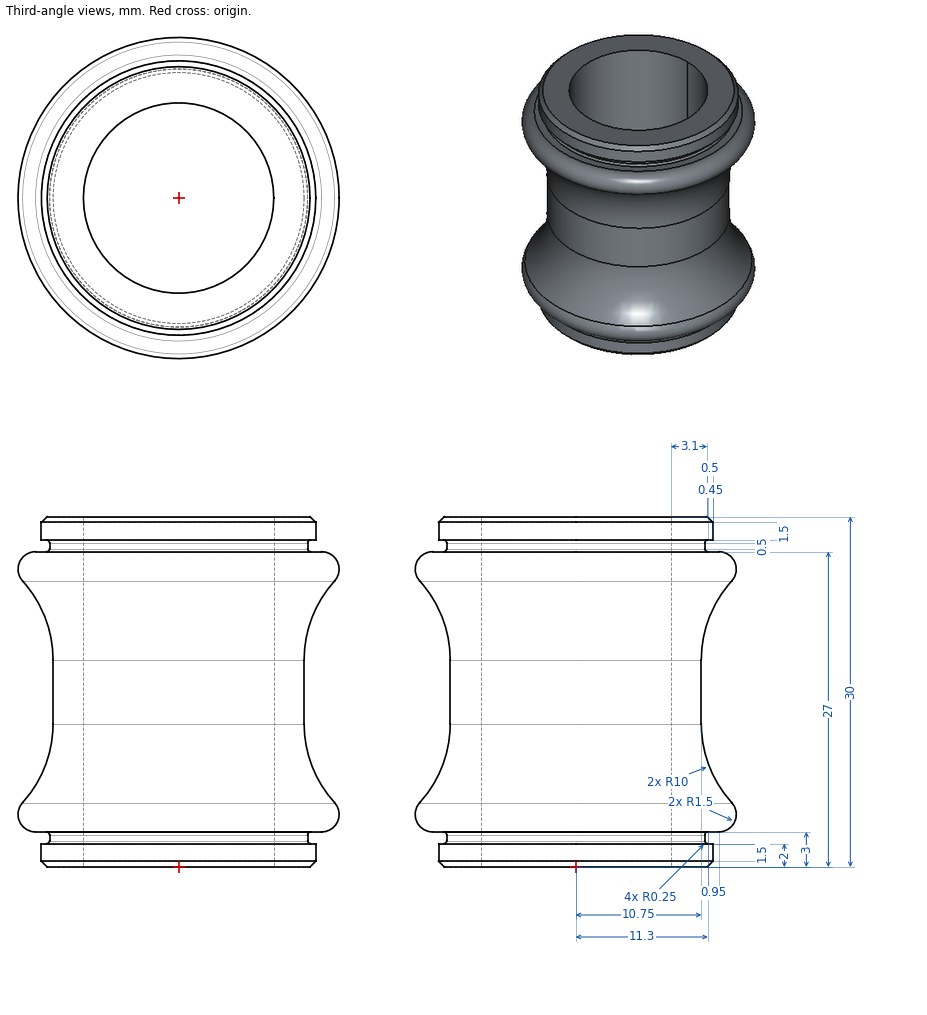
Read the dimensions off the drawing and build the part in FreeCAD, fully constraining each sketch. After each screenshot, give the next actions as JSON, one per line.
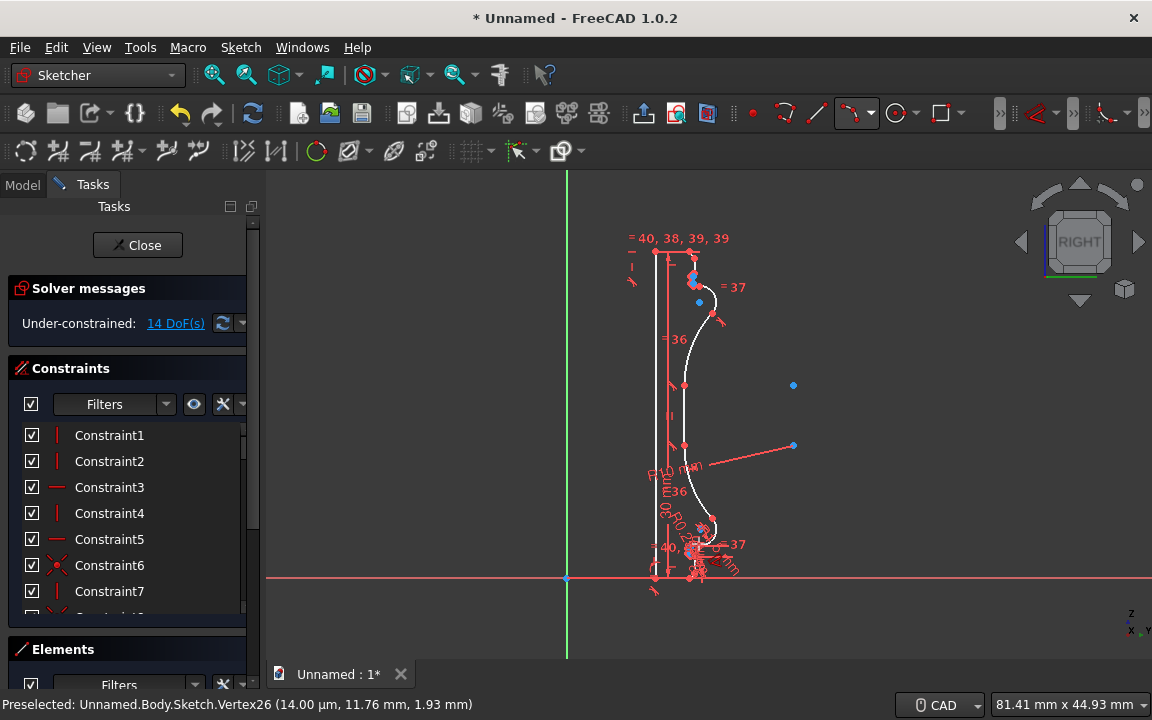
{"action": "scroll", "coordinate": [691, 281], "scroll_direction": "up", "scroll_amount": 10}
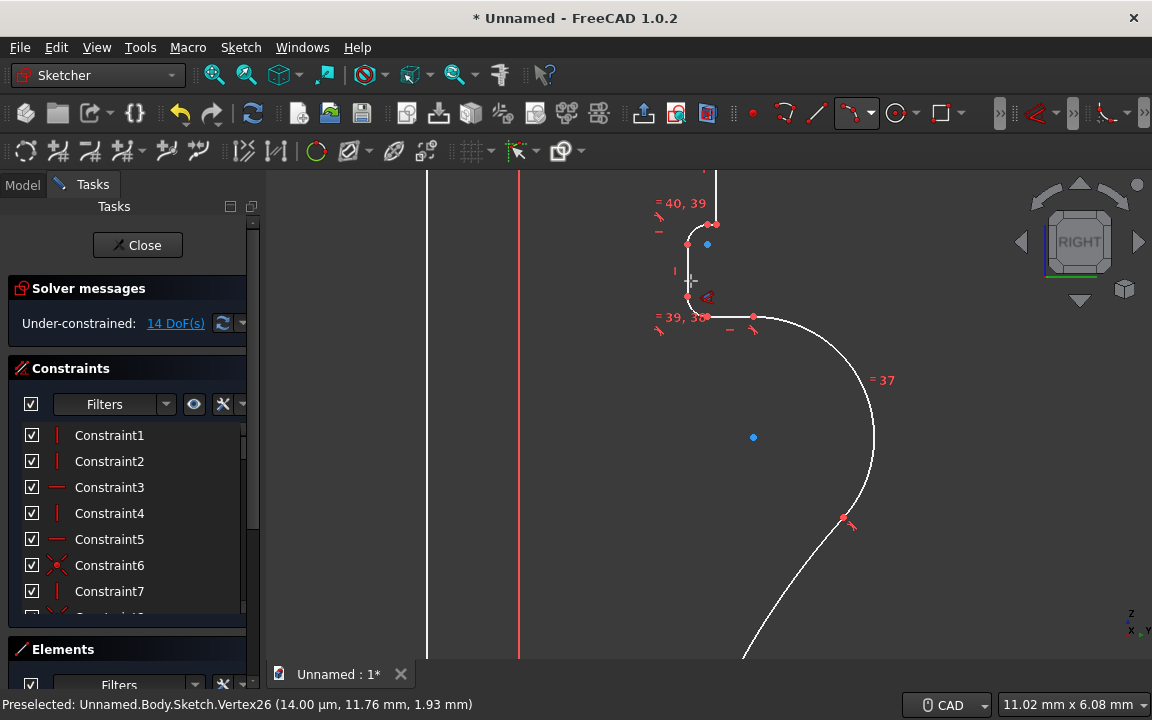
{"action": "left_click", "coordinate": [688, 281]}
{"action": "left_click", "coordinate": [722, 271]}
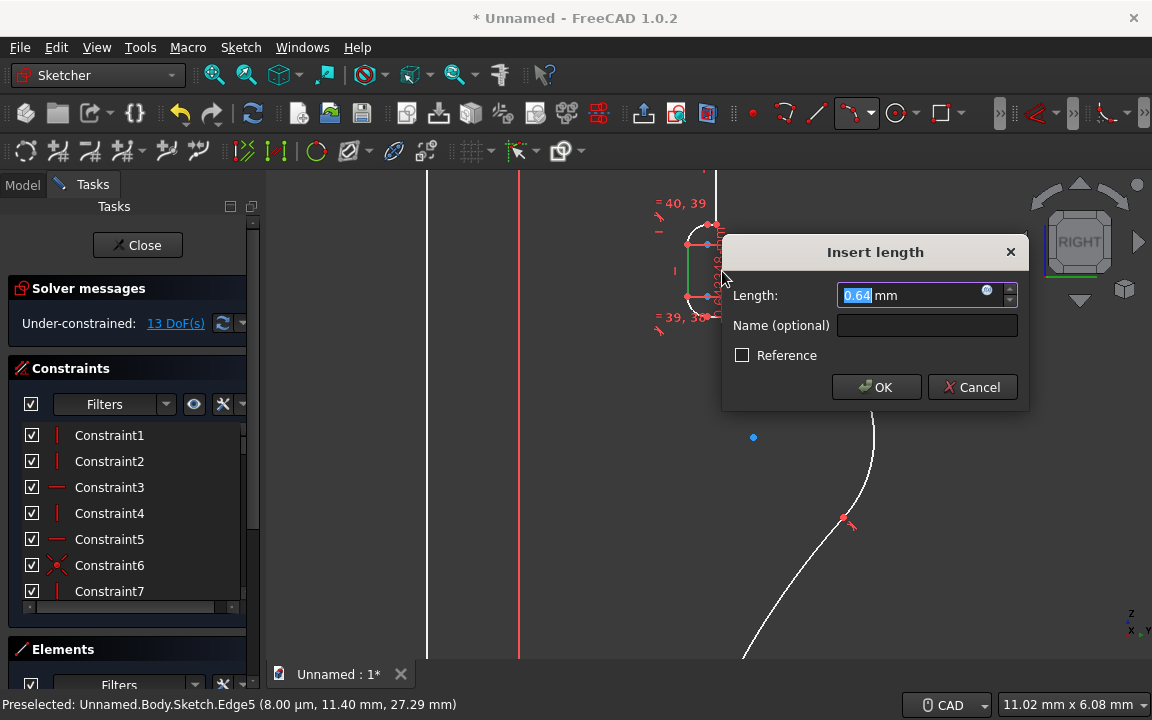
{"action": "type", "text": "0.5"}
{"action": "key", "text": "Return"}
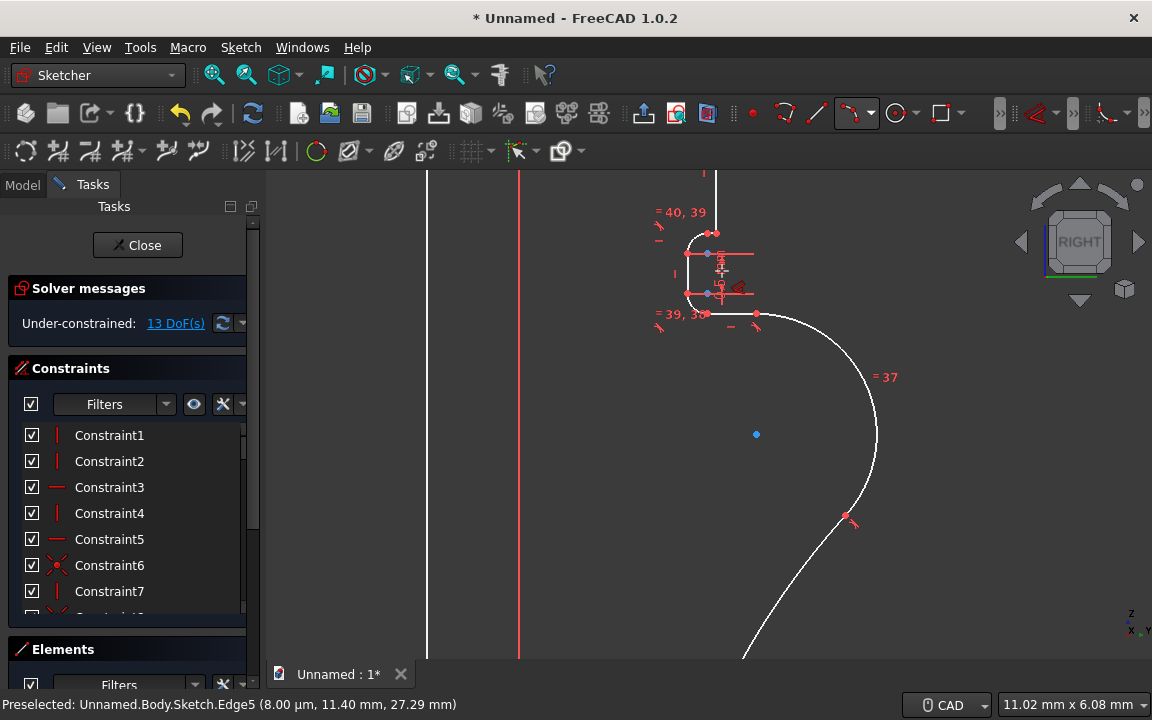
{"action": "left_click", "coordinate": [716, 209]}
{"action": "left_click", "coordinate": [750, 216]}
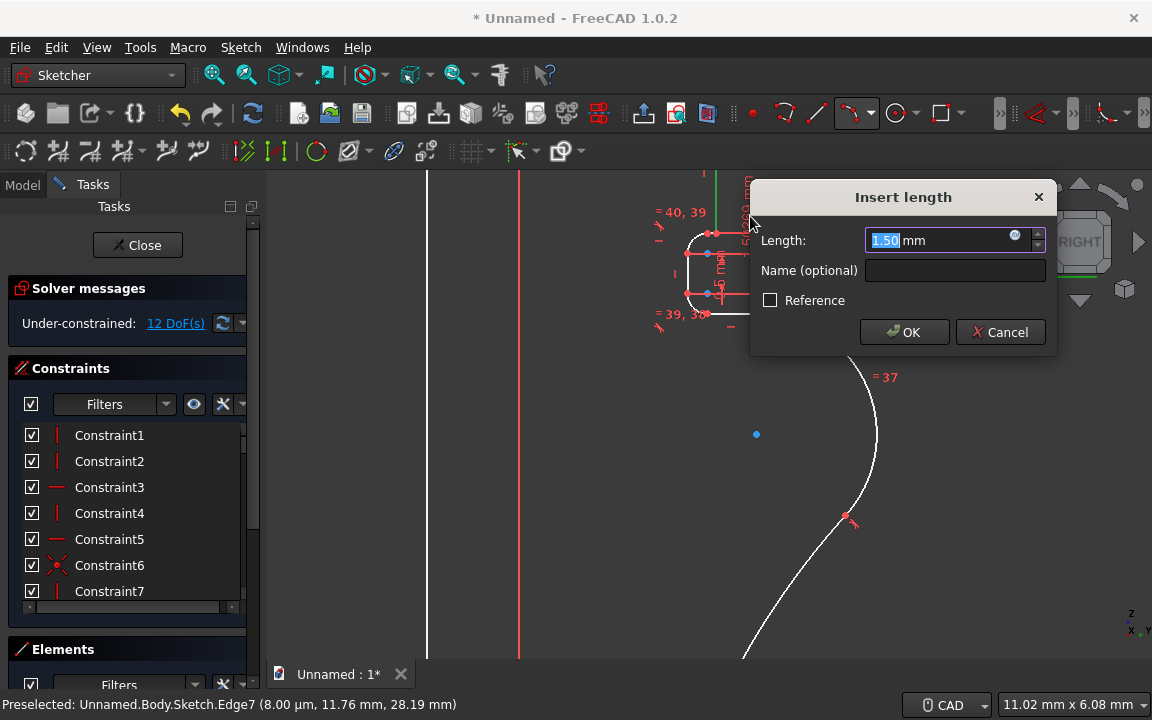
{"action": "type", "text": "1.5"}
{"action": "key", "text": "Return"}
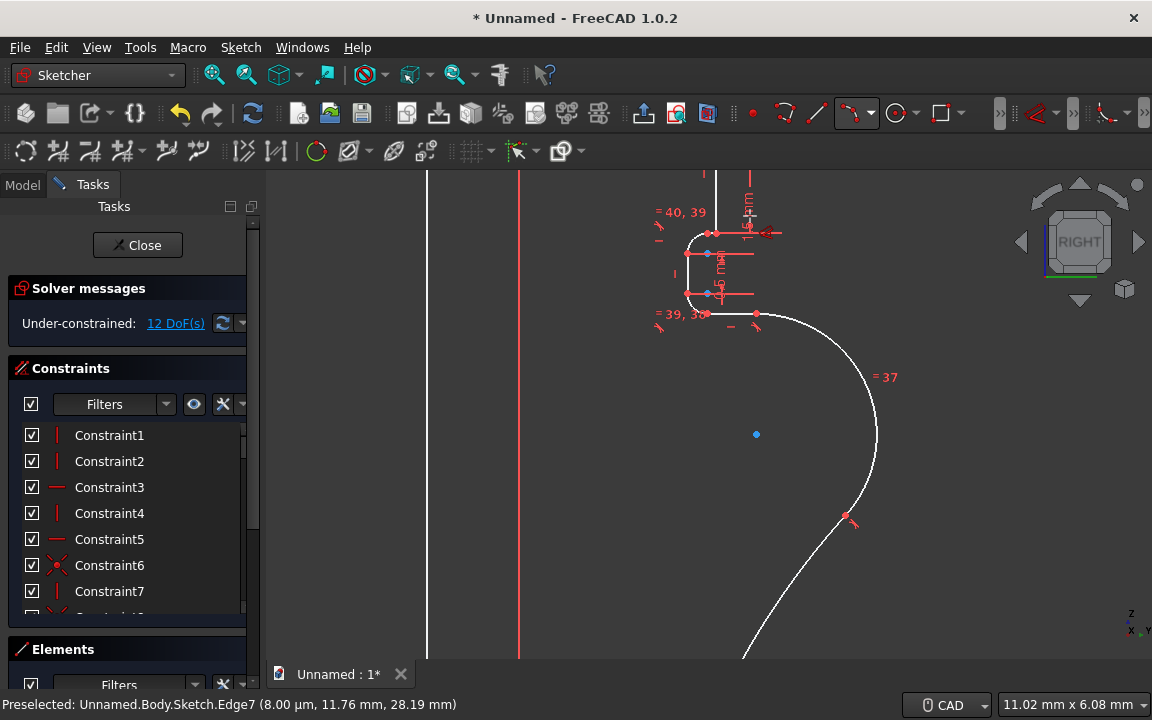
{"action": "scroll", "coordinate": [691, 281], "scroll_direction": "down", "scroll_amount": 10}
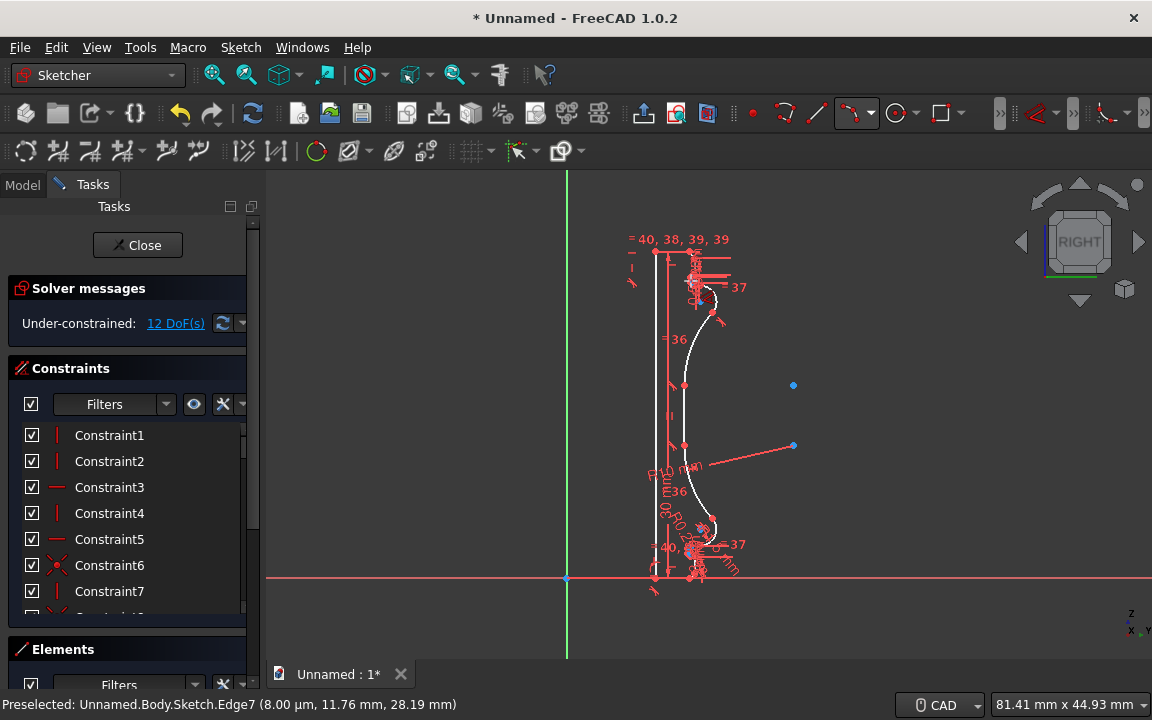
{"action": "scroll", "coordinate": [679, 252], "scroll_direction": "up", "scroll_amount": 2}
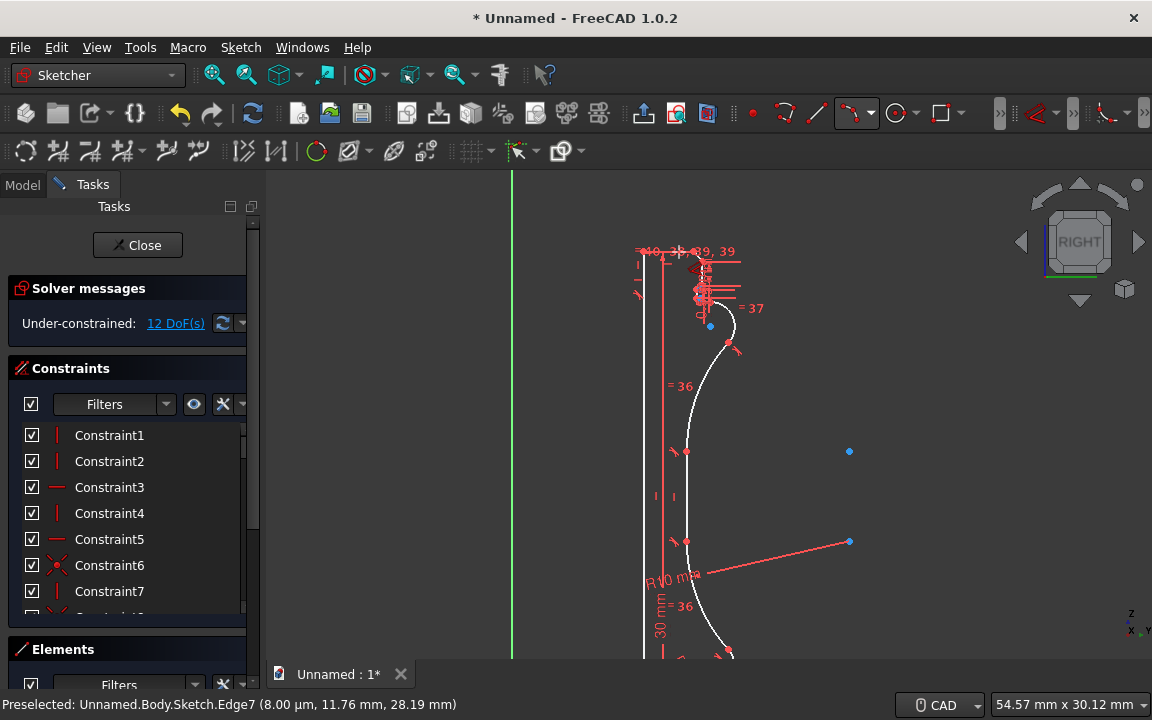
{"action": "left_click", "coordinate": [679, 252]}
{"action": "left_click", "coordinate": [669, 218]}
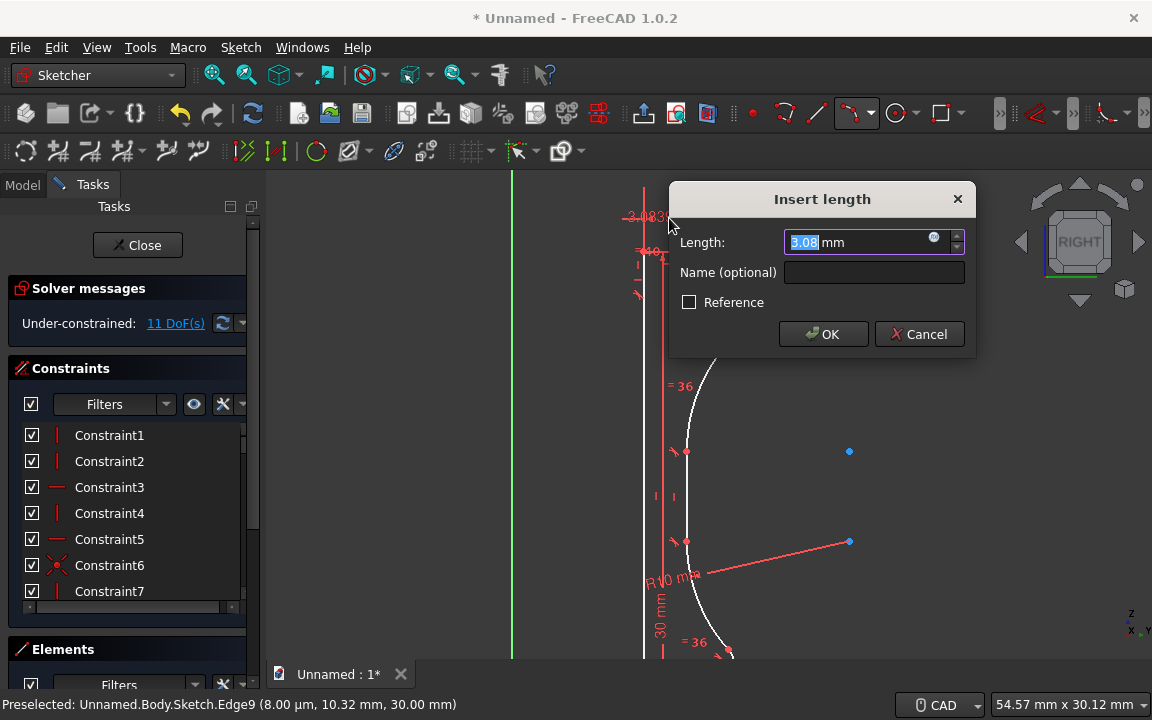
{"action": "type", "text": "3.1"}
{"action": "key", "text": "Return"}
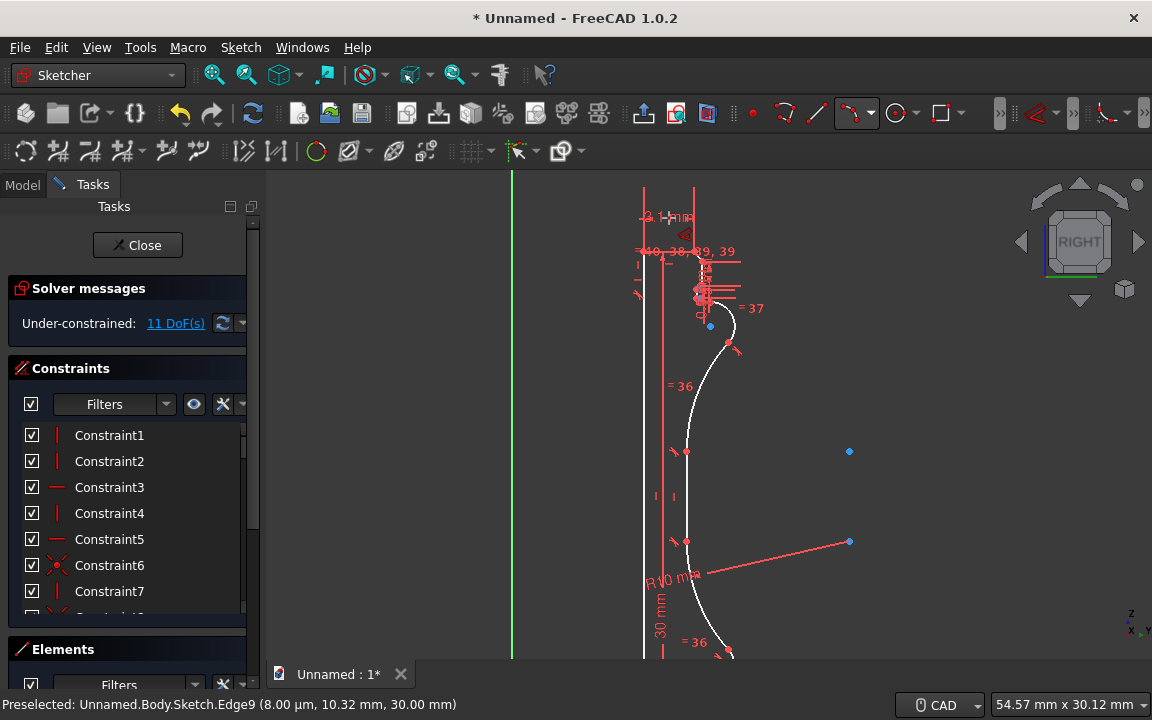
{"action": "scroll", "coordinate": [678, 250], "scroll_direction": "down", "scroll_amount": 2}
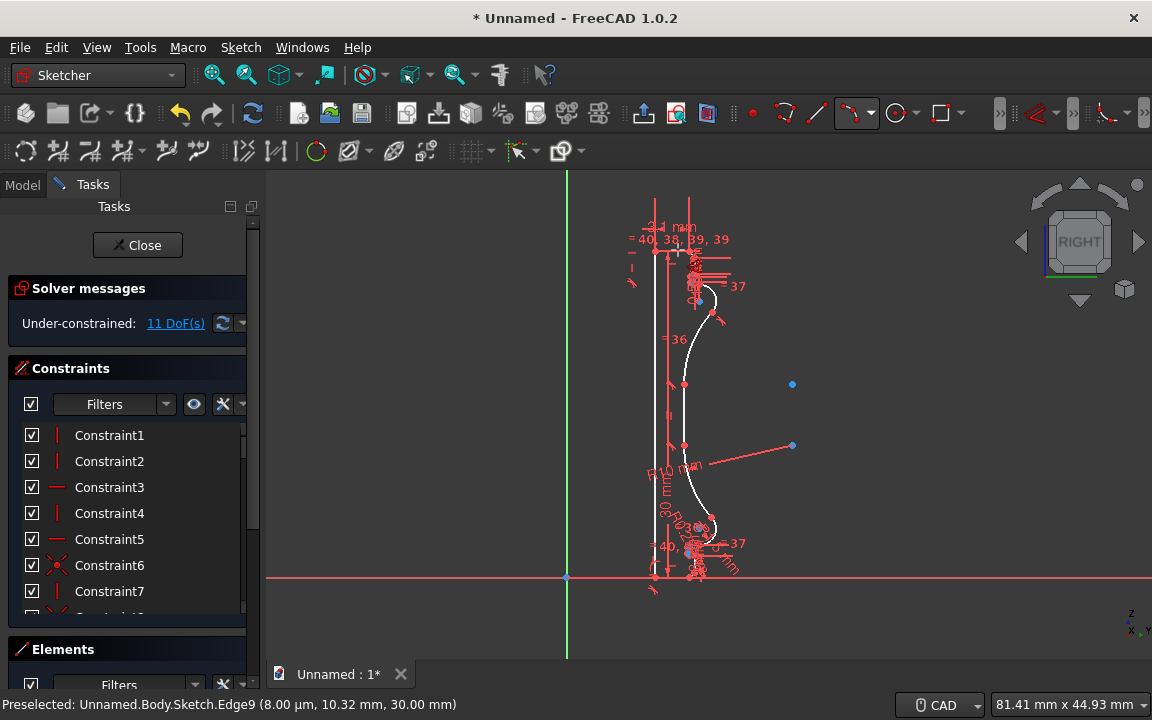
{"action": "scroll", "coordinate": [666, 578], "scroll_direction": "up", "scroll_amount": 2}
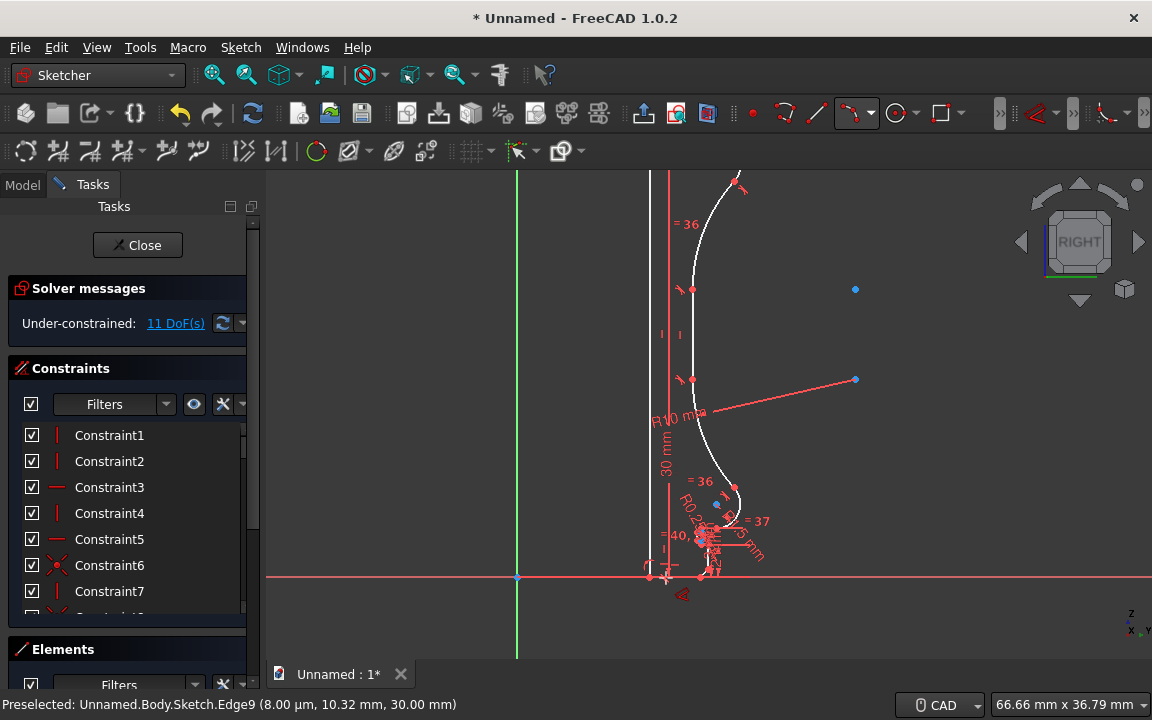
{"action": "left_click", "coordinate": [665, 577]}
{"action": "left_click", "coordinate": [675, 611]}